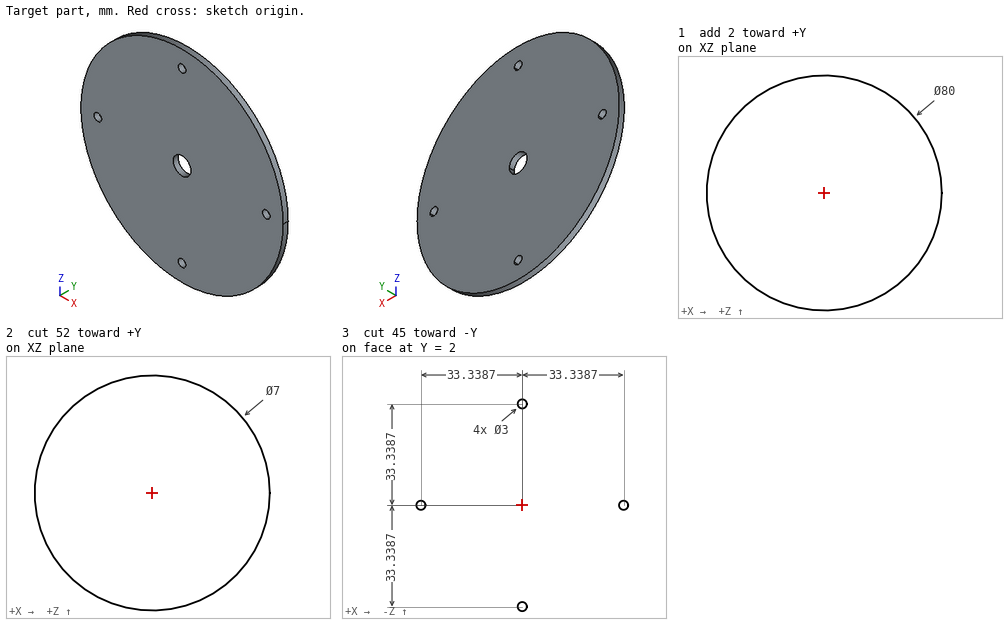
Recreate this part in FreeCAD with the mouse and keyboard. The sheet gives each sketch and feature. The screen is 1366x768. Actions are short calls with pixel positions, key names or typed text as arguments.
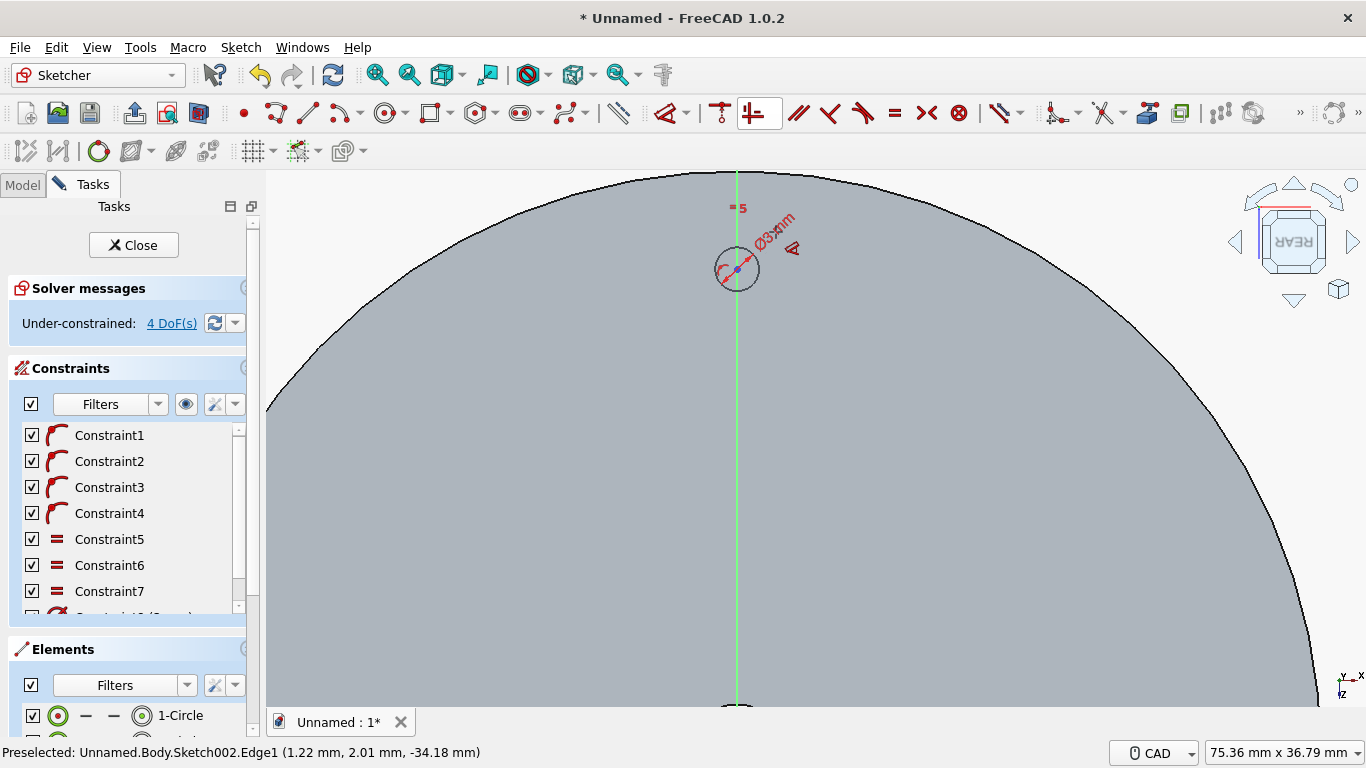
click(737, 269)
click(771, 474)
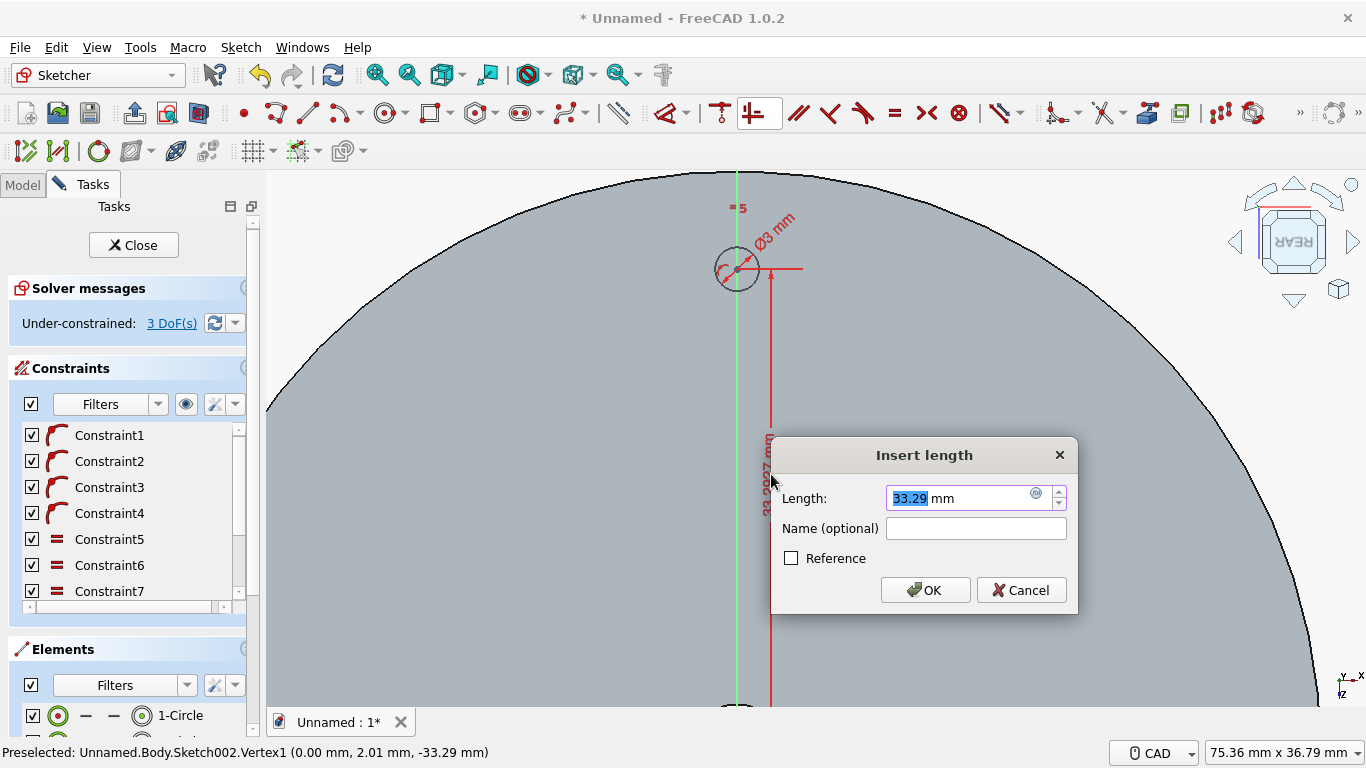
text(33.3387)
key(Return)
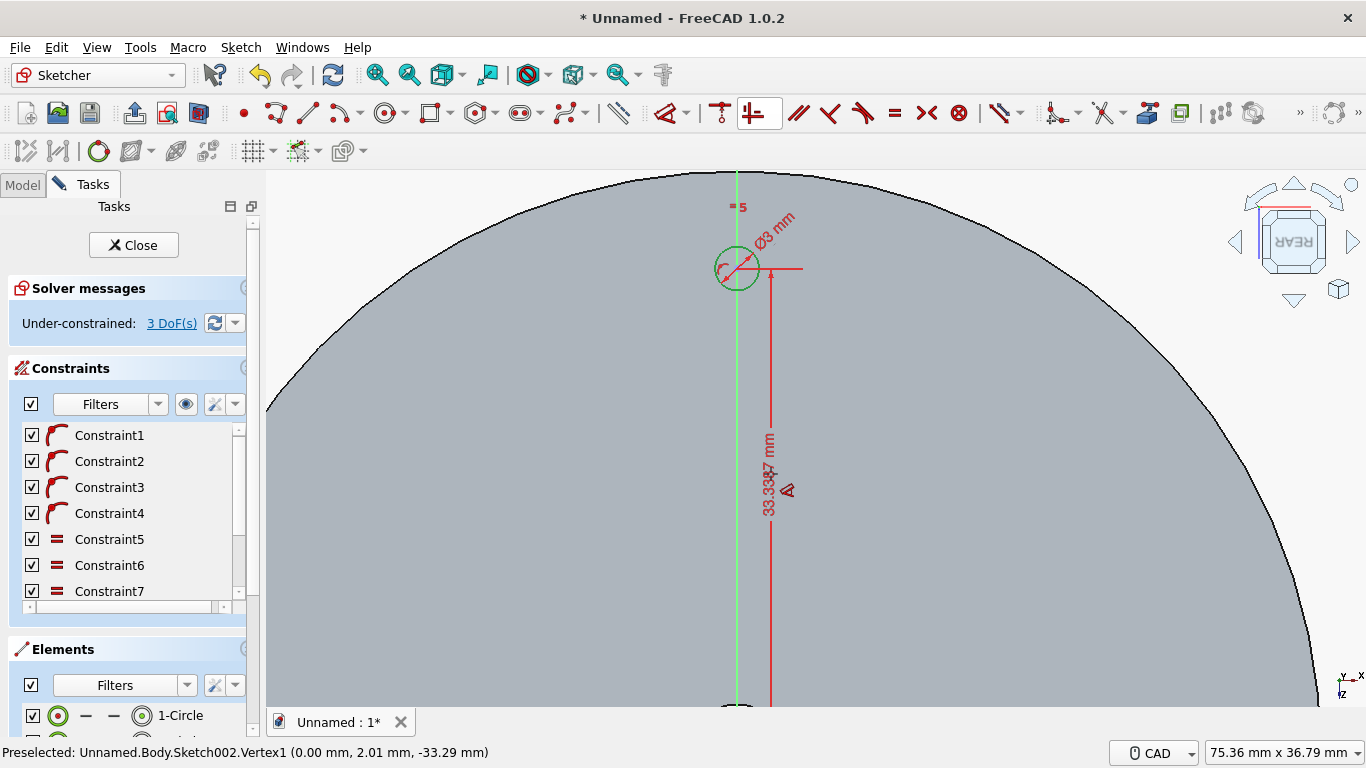
scroll(754, 254, down, 5)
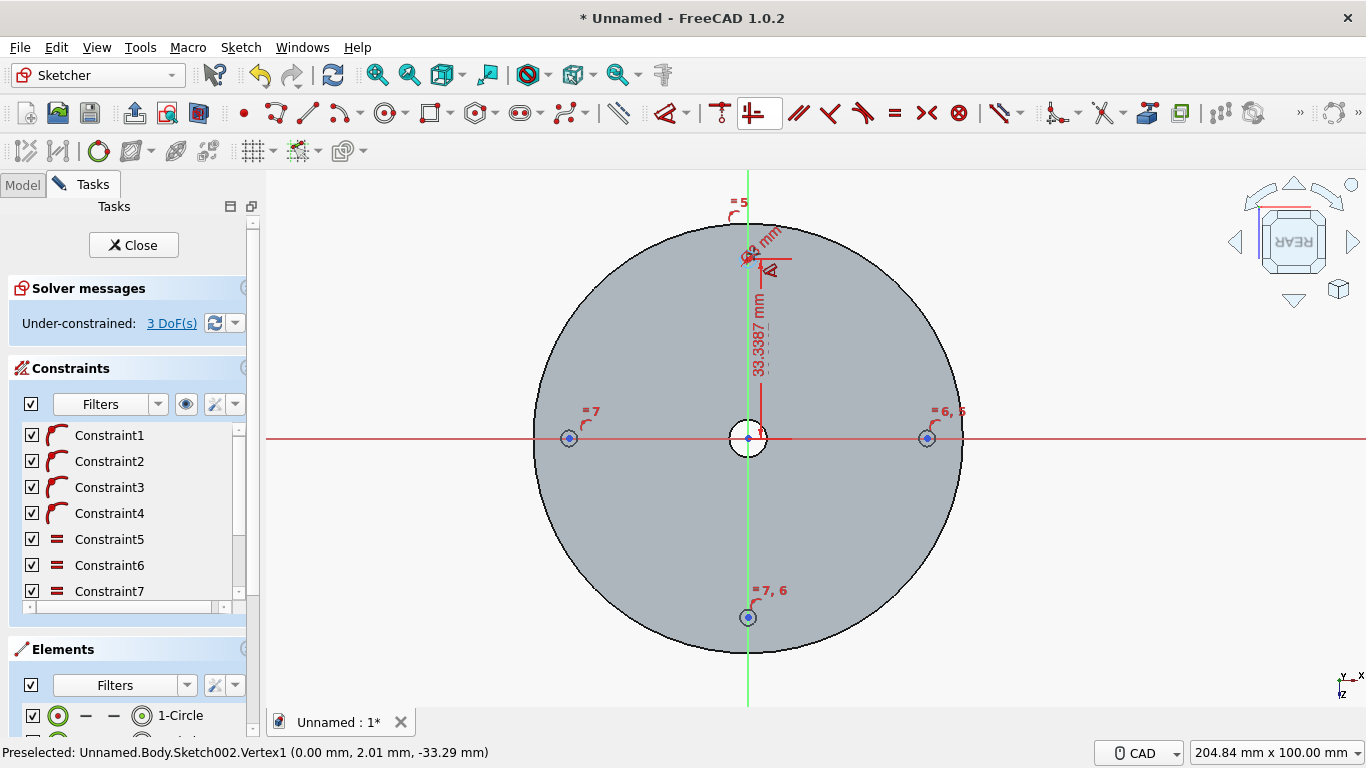
click(927, 439)
click(838, 473)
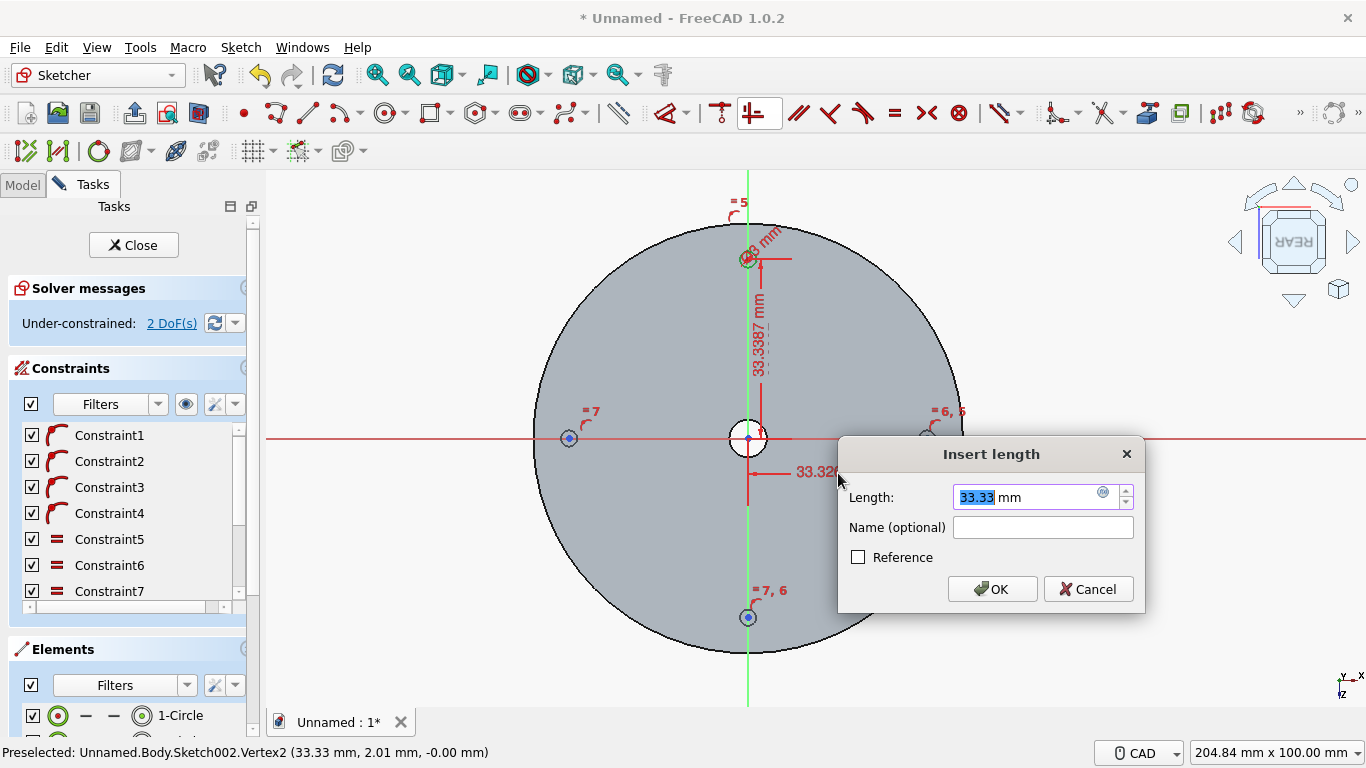
text(33.3387)
key(Return)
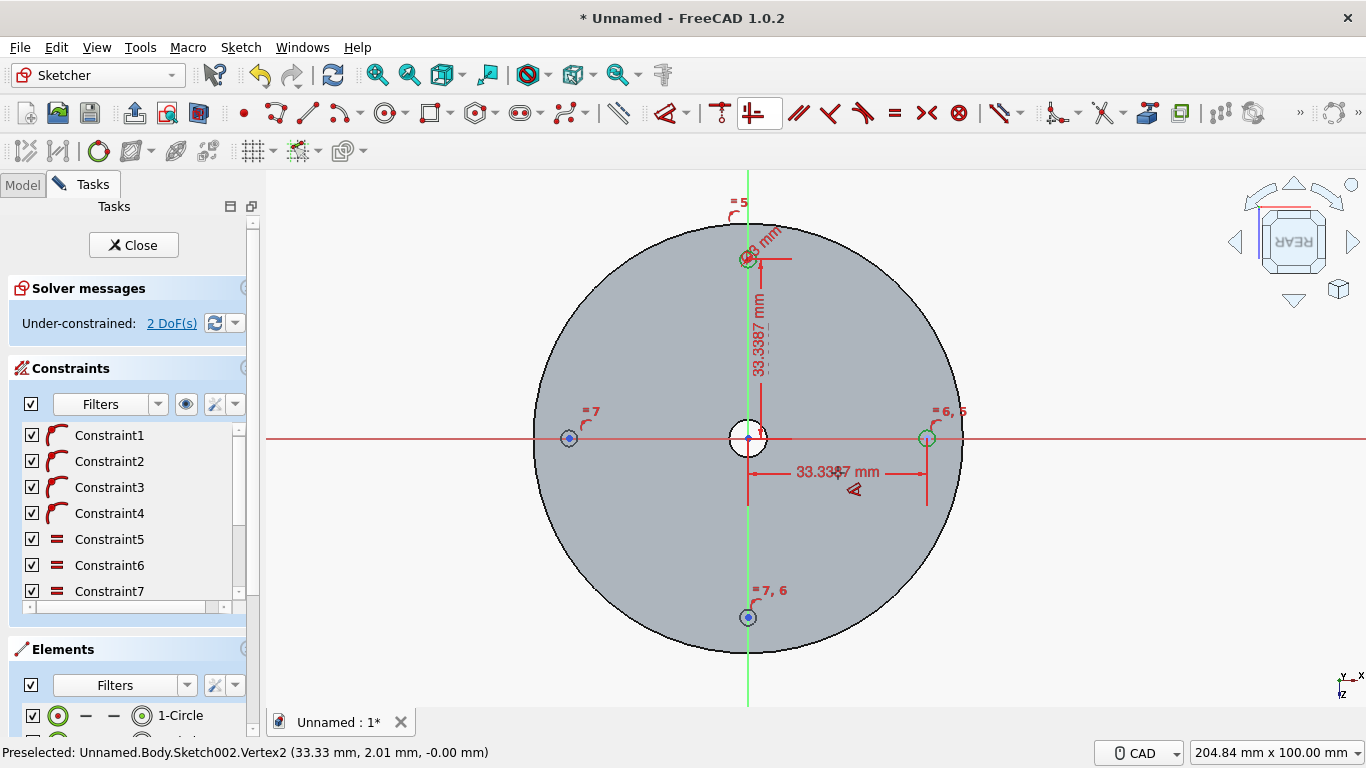
click(748, 618)
click(782, 528)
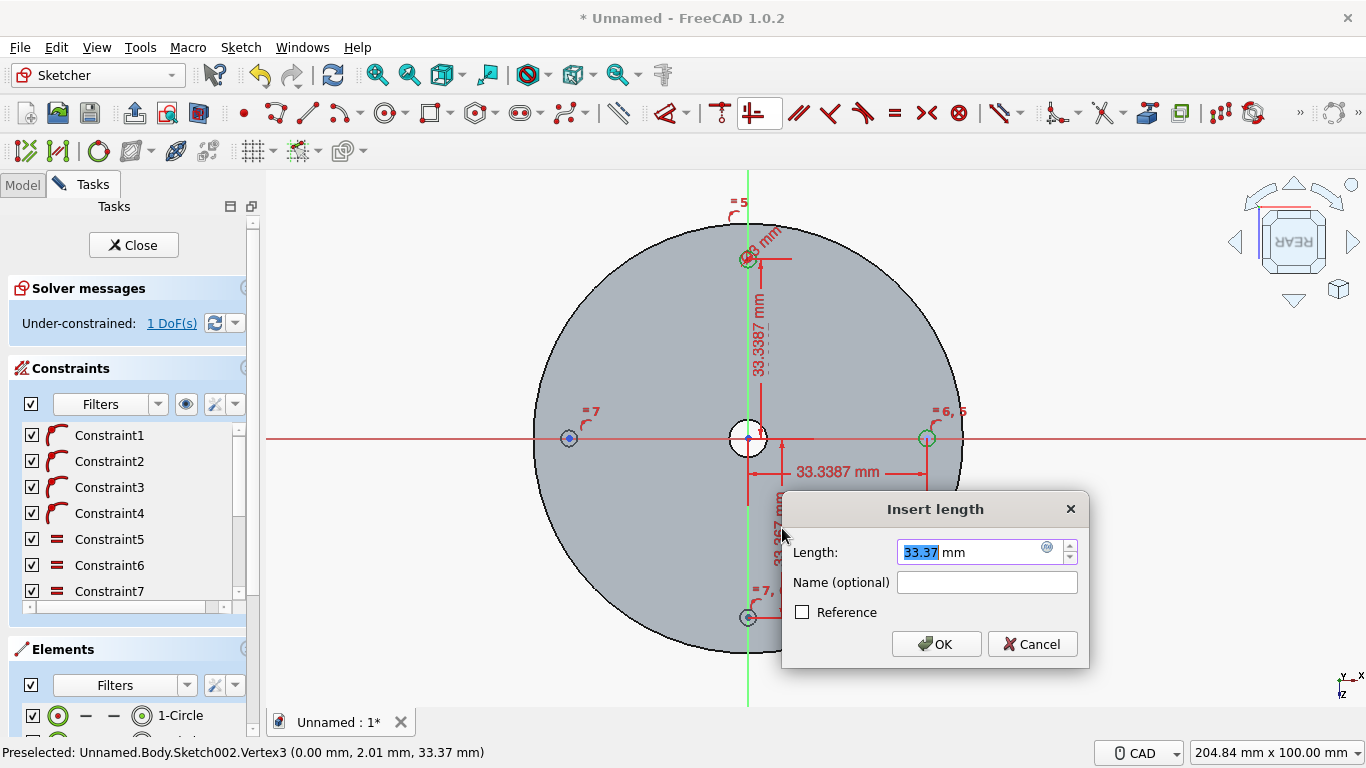
text(33.3387)
key(Return)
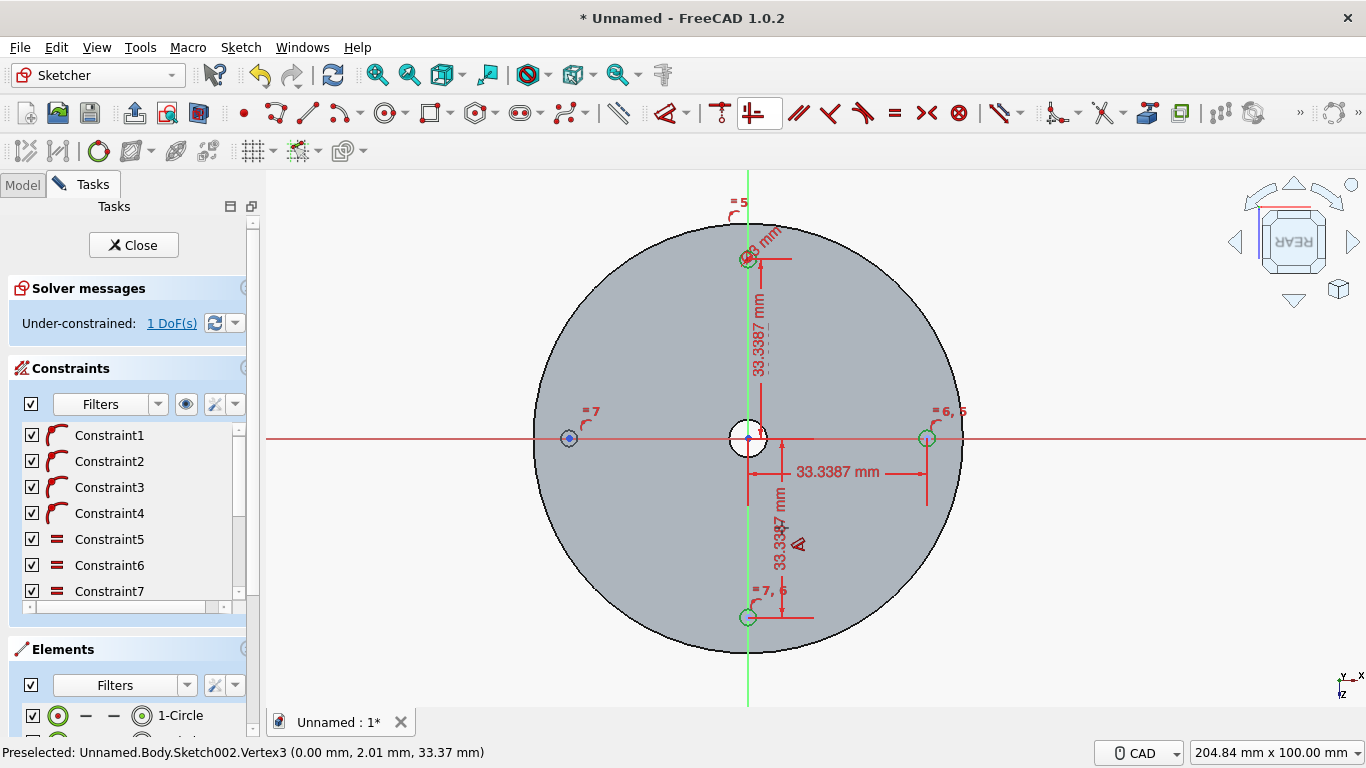
click(569, 439)
click(659, 473)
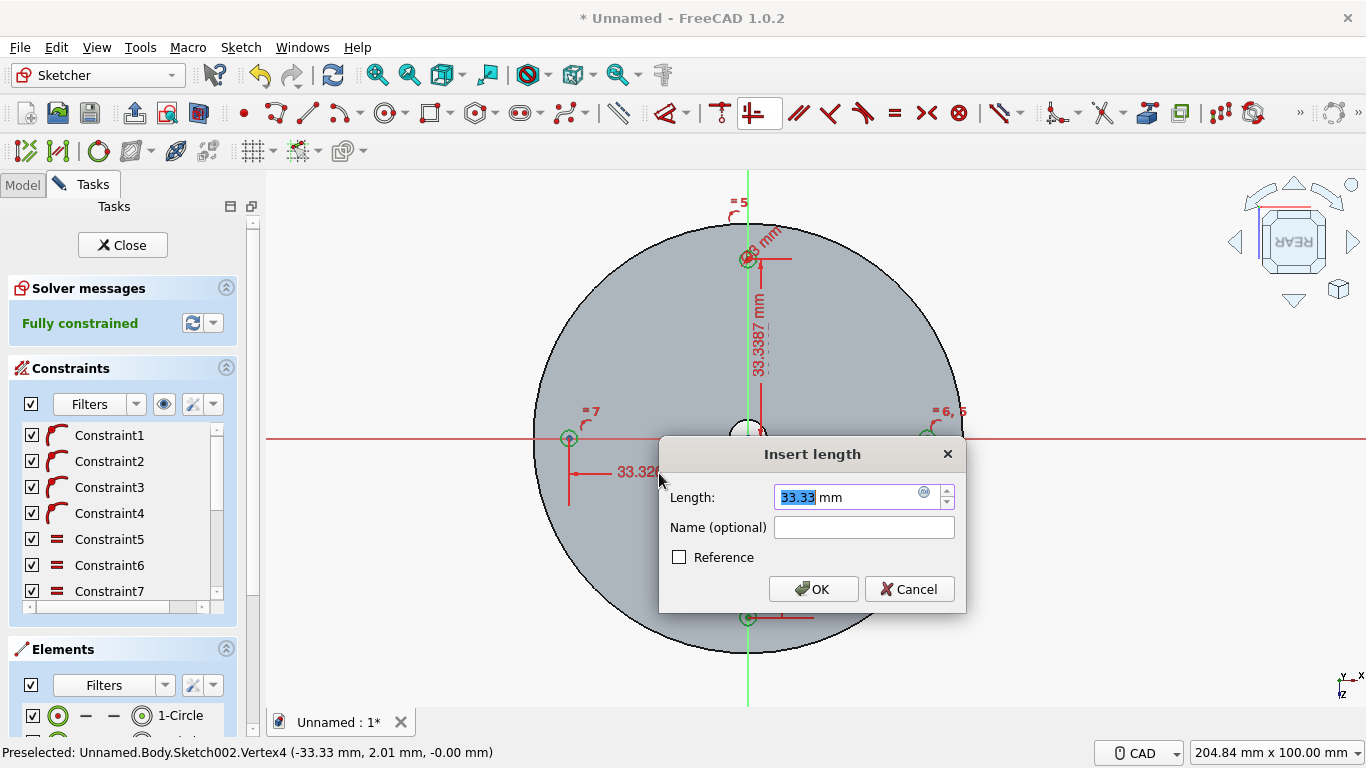
text(33.3387)
key(Return)
key(Escape)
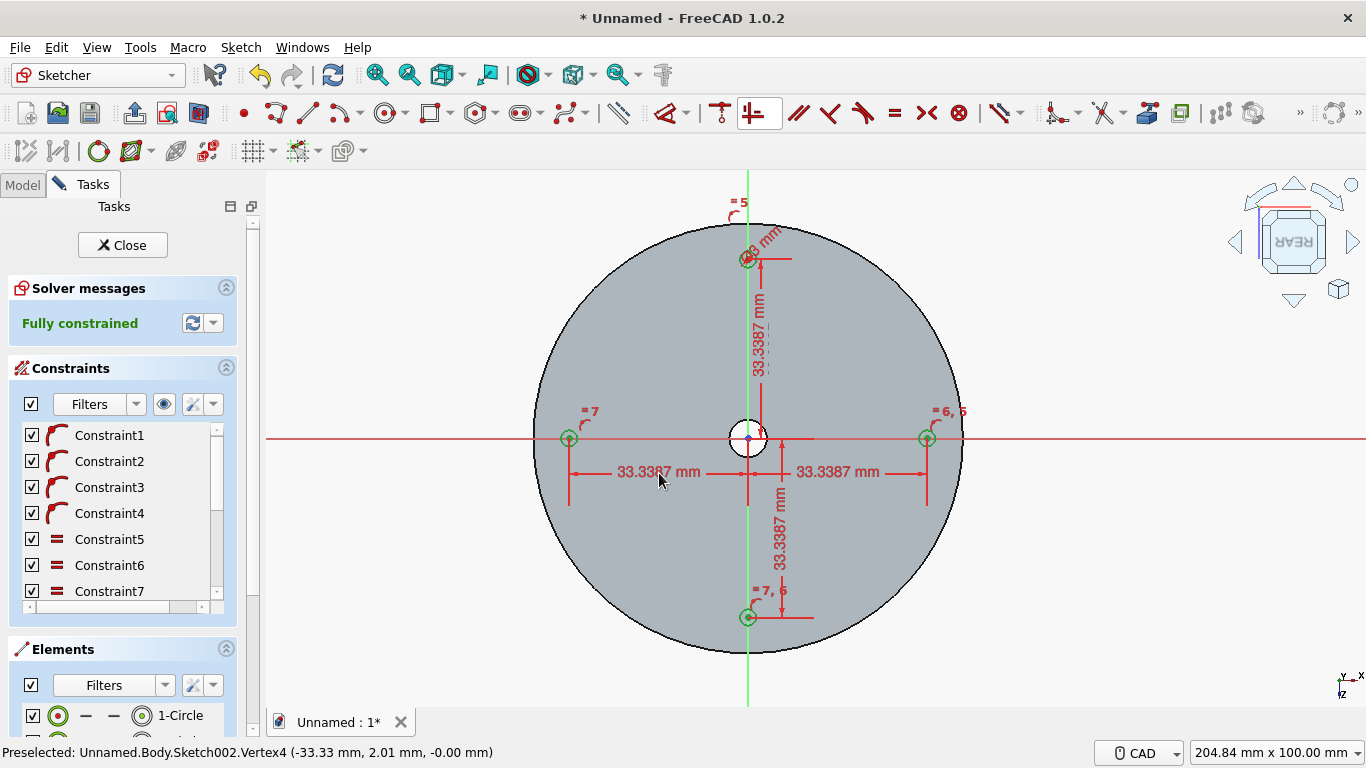
click(123, 245)